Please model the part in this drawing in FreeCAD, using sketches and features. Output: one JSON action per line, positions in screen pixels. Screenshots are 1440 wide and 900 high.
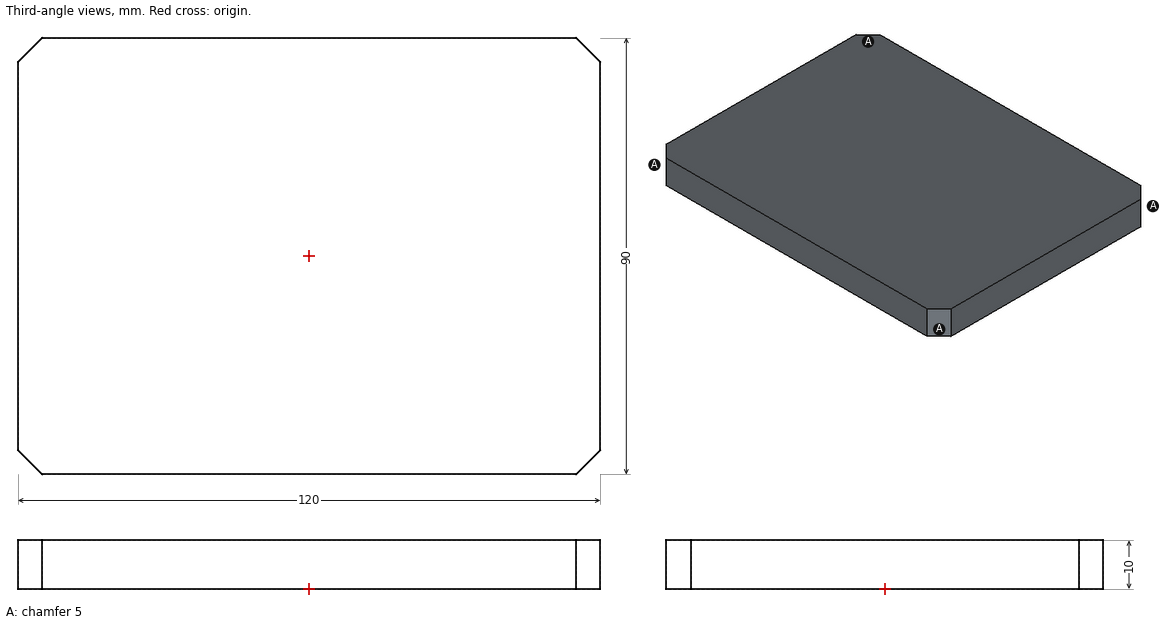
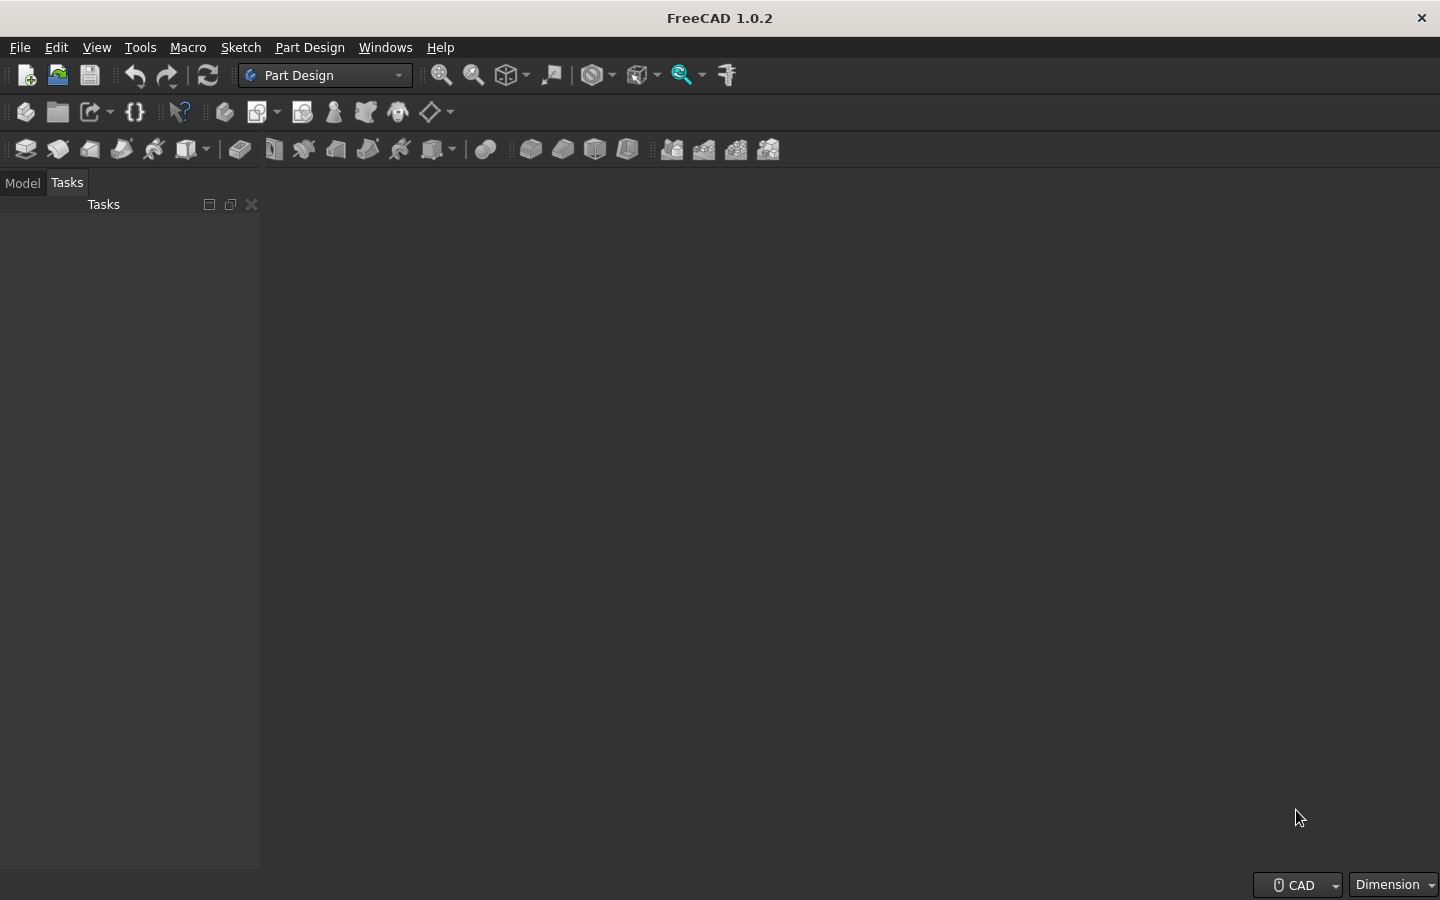
{"action": "left_click", "coordinate": [26, 76]}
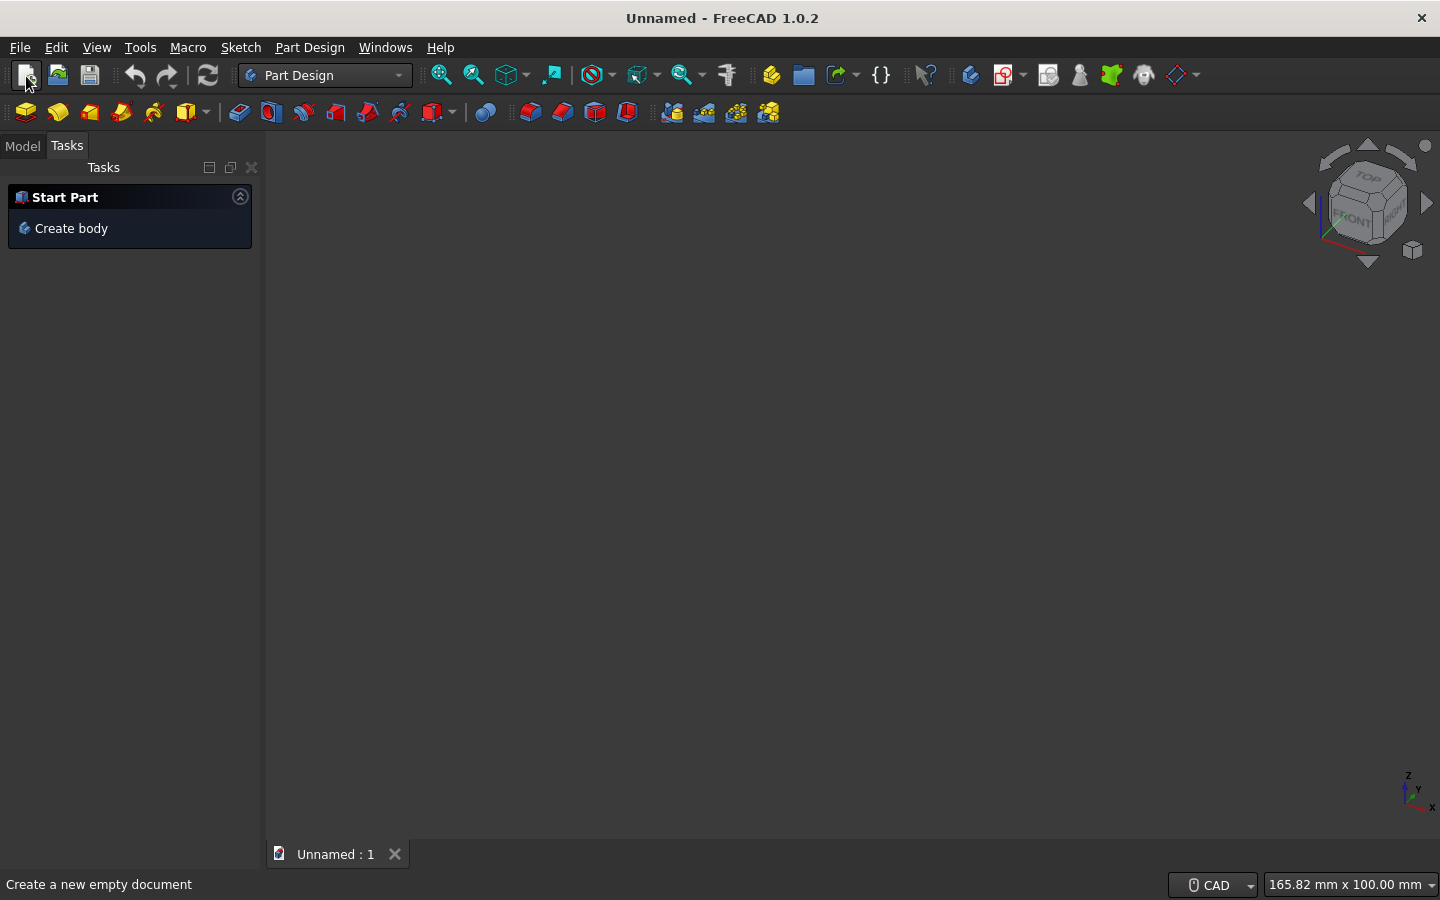
{"action": "left_click", "coordinate": [1004, 76]}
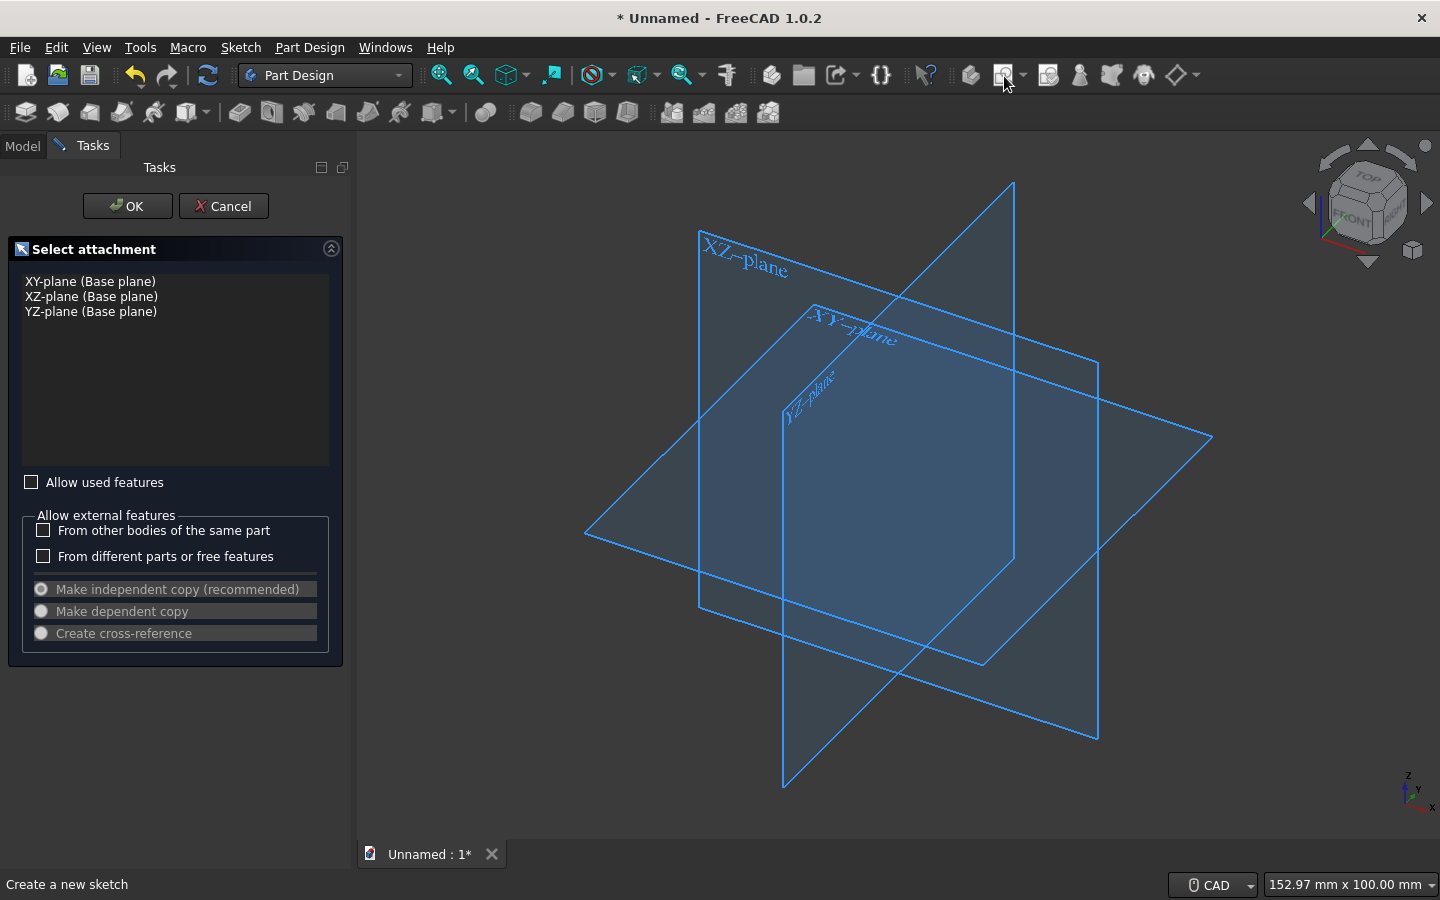
{"action": "left_click", "coordinate": [82, 282]}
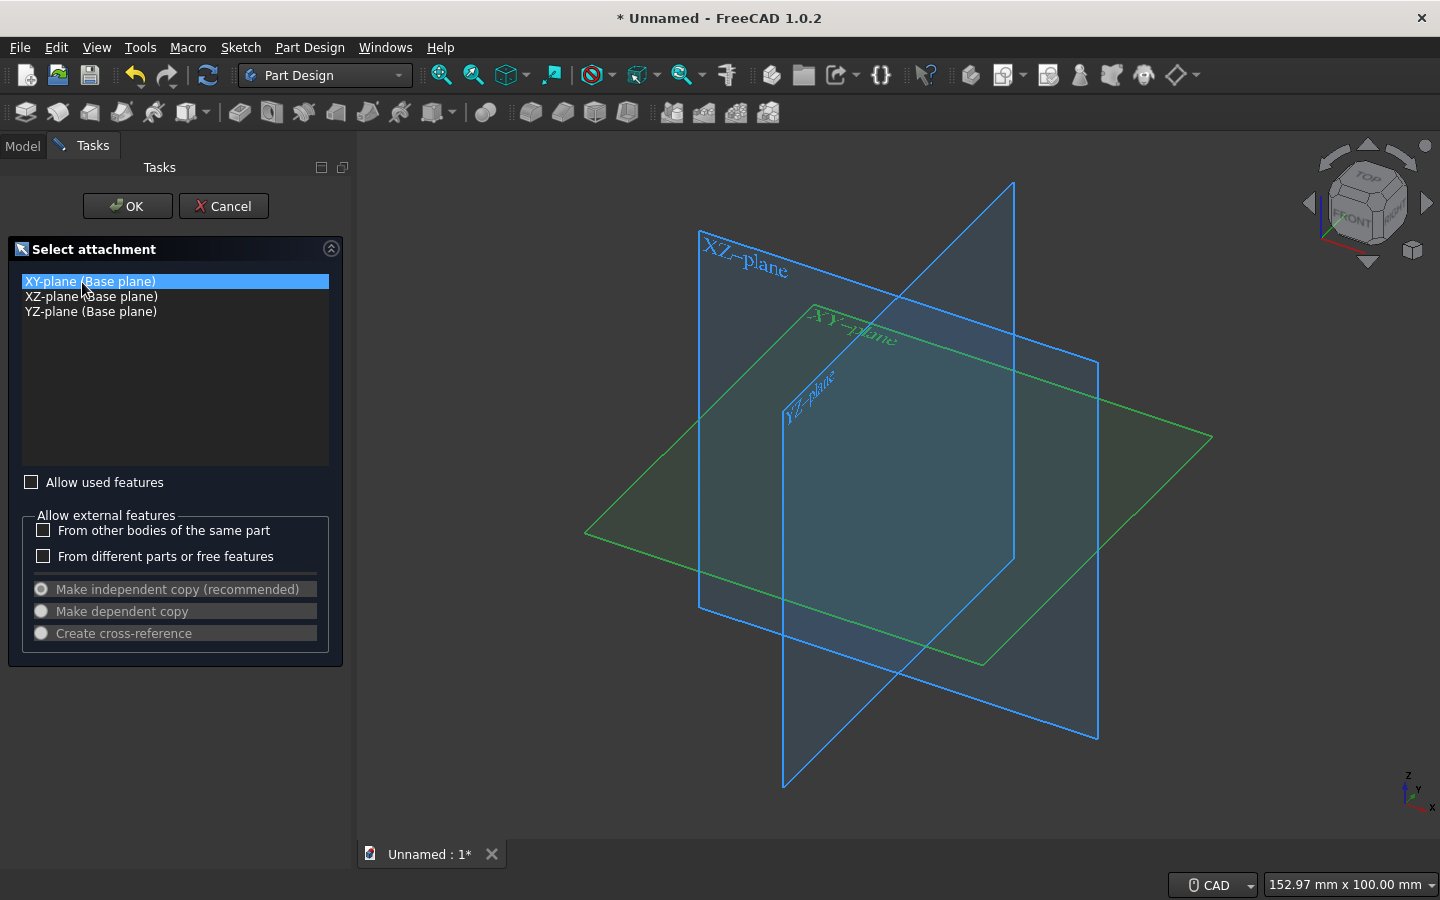
{"action": "left_click", "coordinate": [128, 206]}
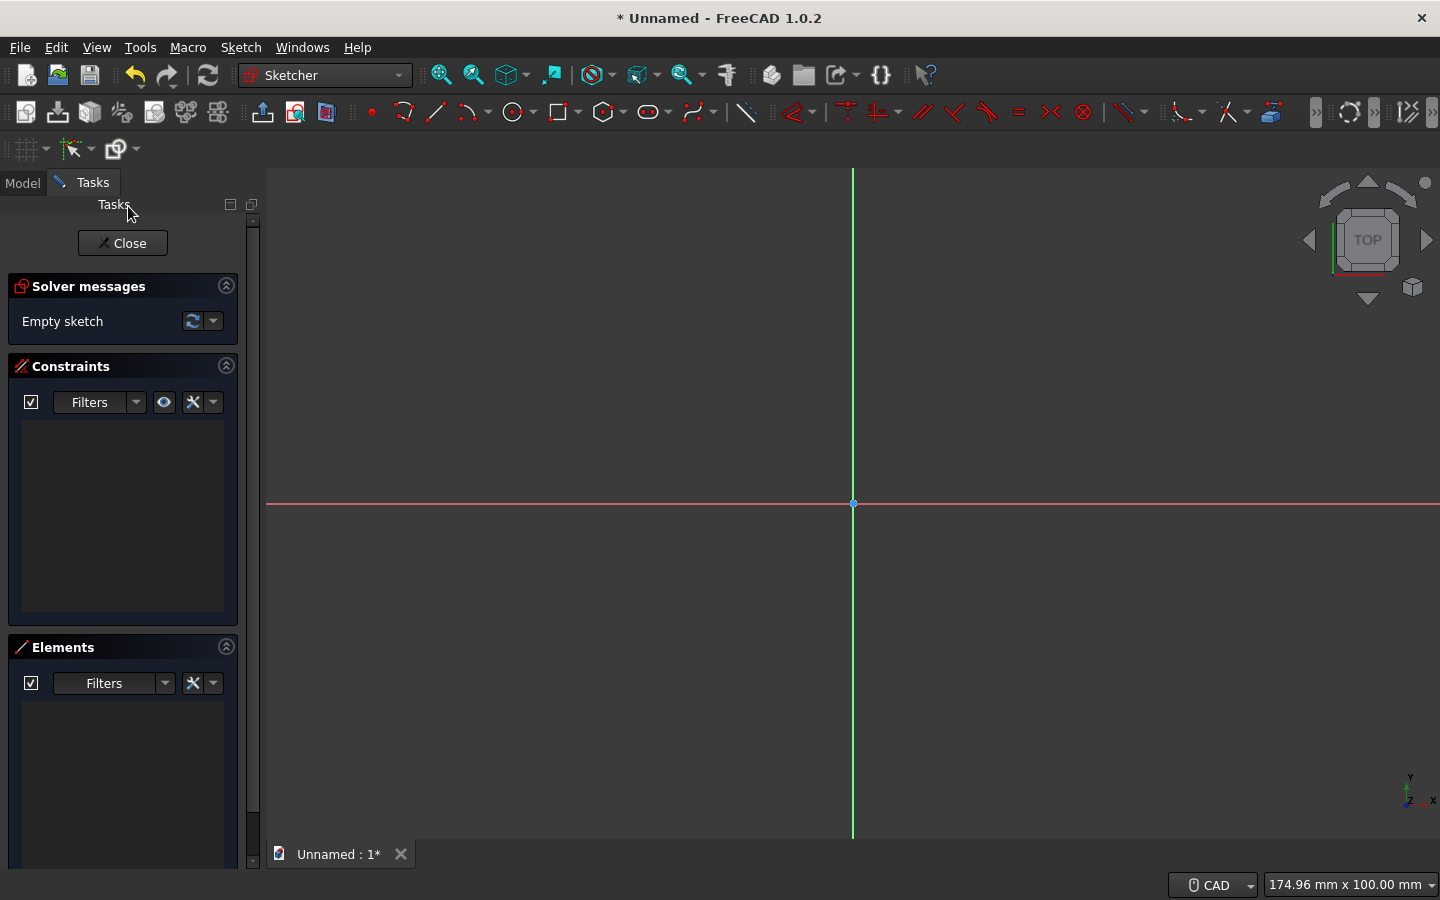
{"action": "scroll", "coordinate": [645, 504], "scroll_direction": "down", "scroll_amount": 2}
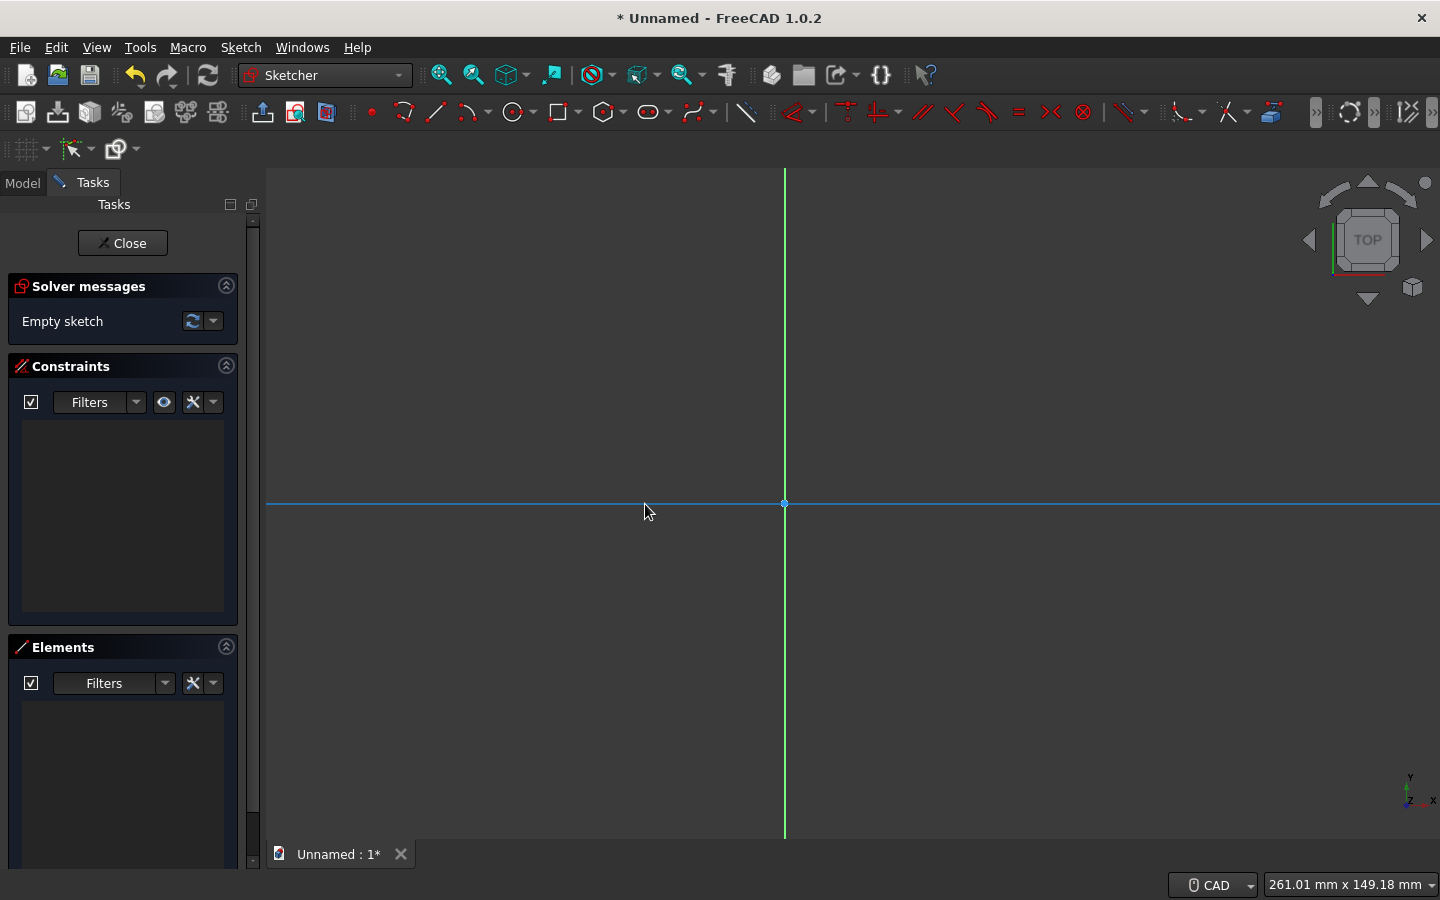
{"action": "key", "text": "g v"}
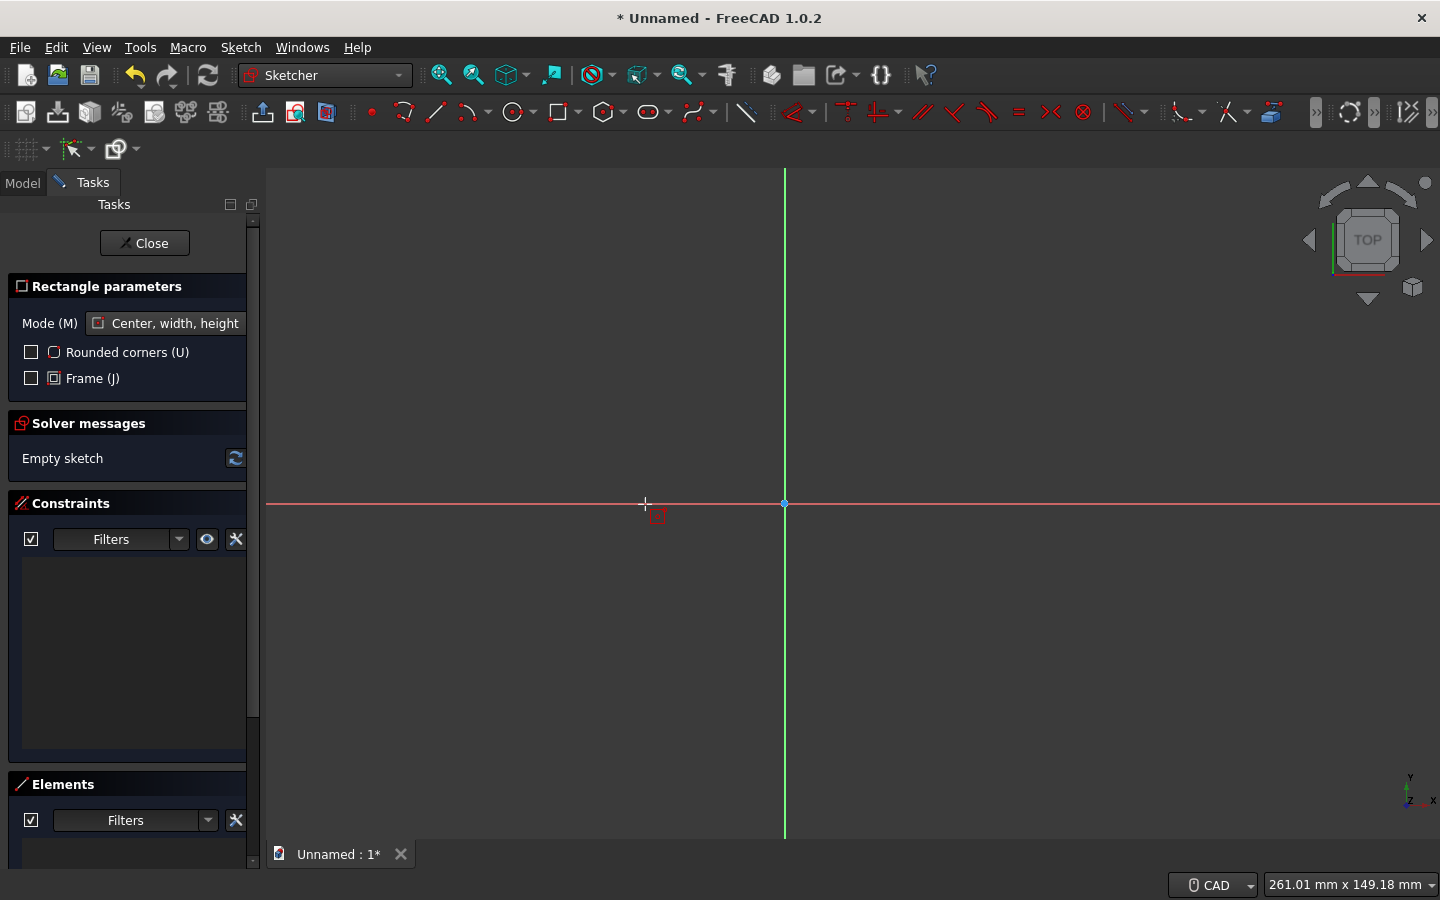
{"action": "left_click", "coordinate": [785, 504]}
{"action": "left_click", "coordinate": [1054, 301]}
{"action": "key", "text": "Escape"}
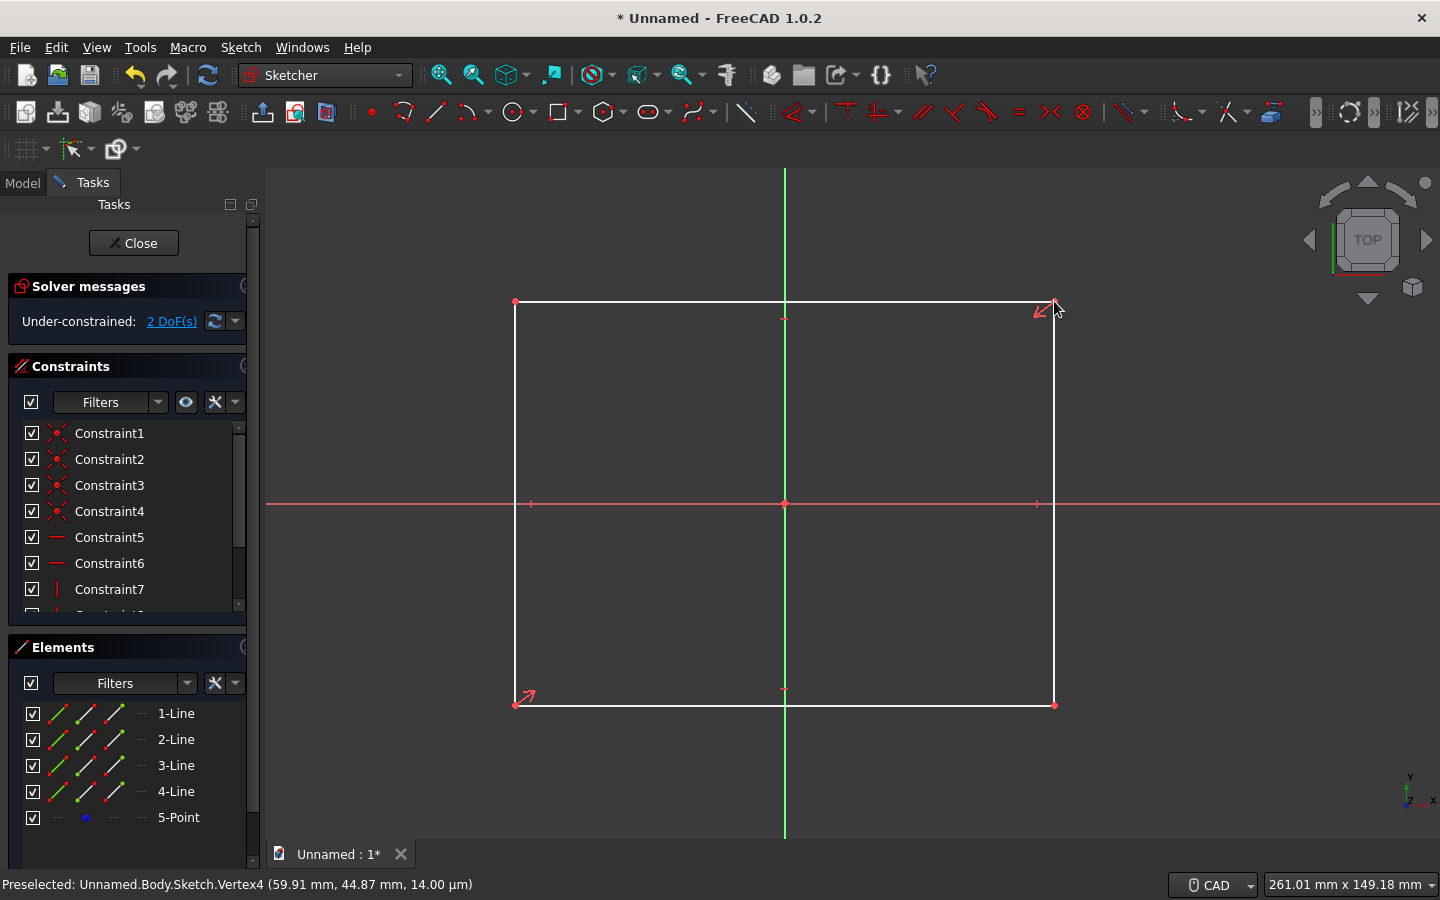
{"action": "left_click", "coordinate": [792, 112]}